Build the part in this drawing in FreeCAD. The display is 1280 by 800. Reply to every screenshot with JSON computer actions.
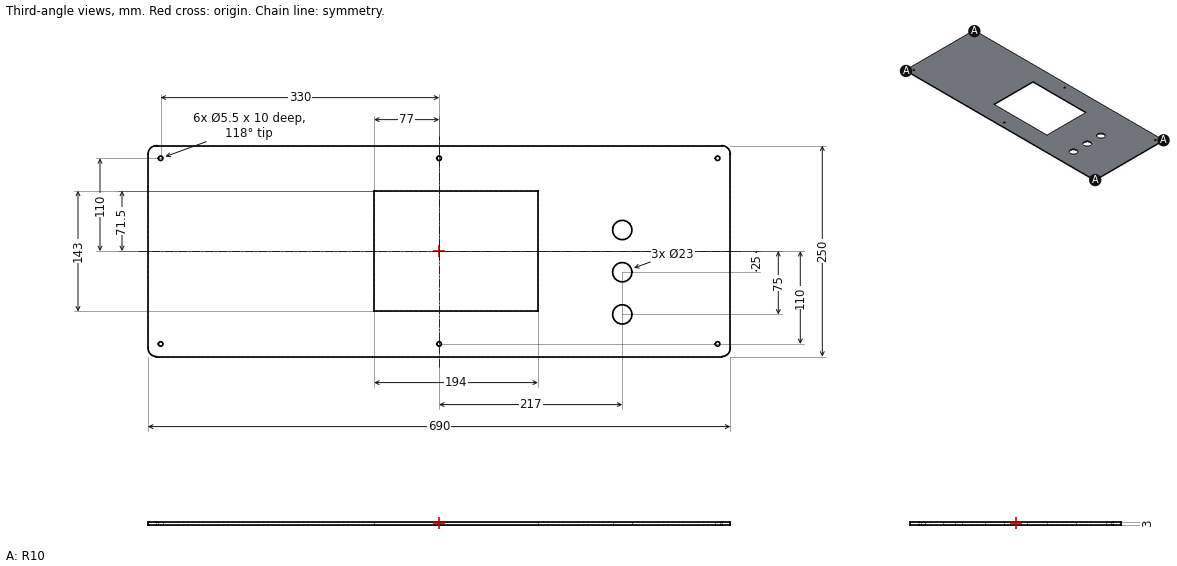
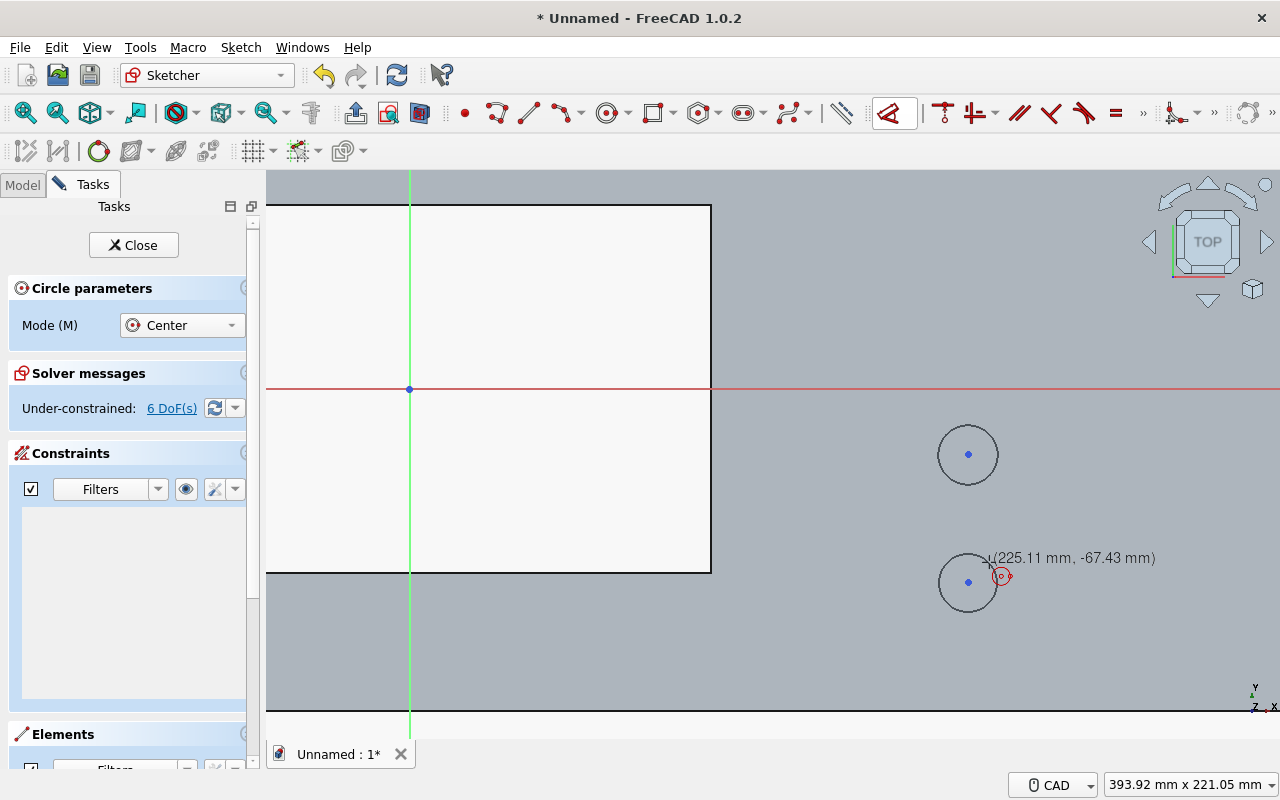
{"action": "left_click", "coordinate": [968, 325]}
{"action": "left_click", "coordinate": [989, 304]}
{"action": "key", "text": "Escape"}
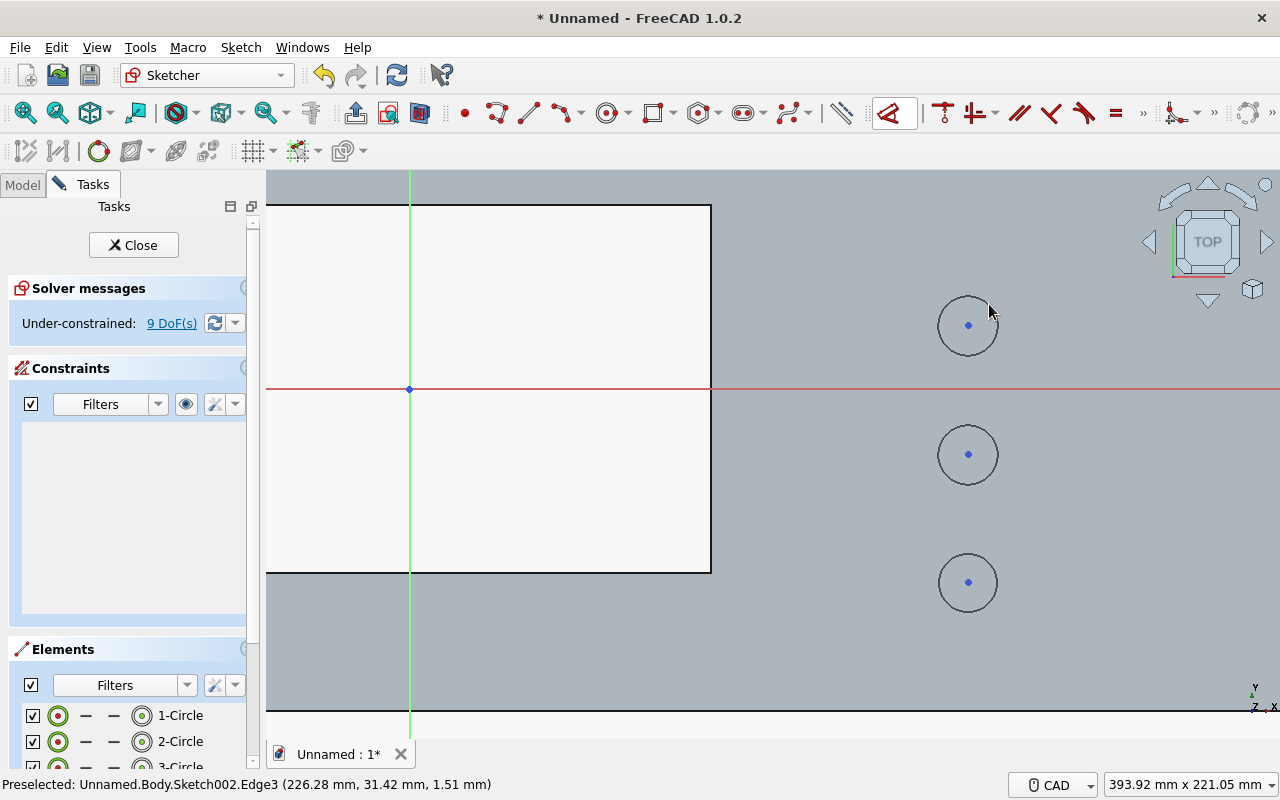
{"action": "left_click", "coordinate": [989, 434]}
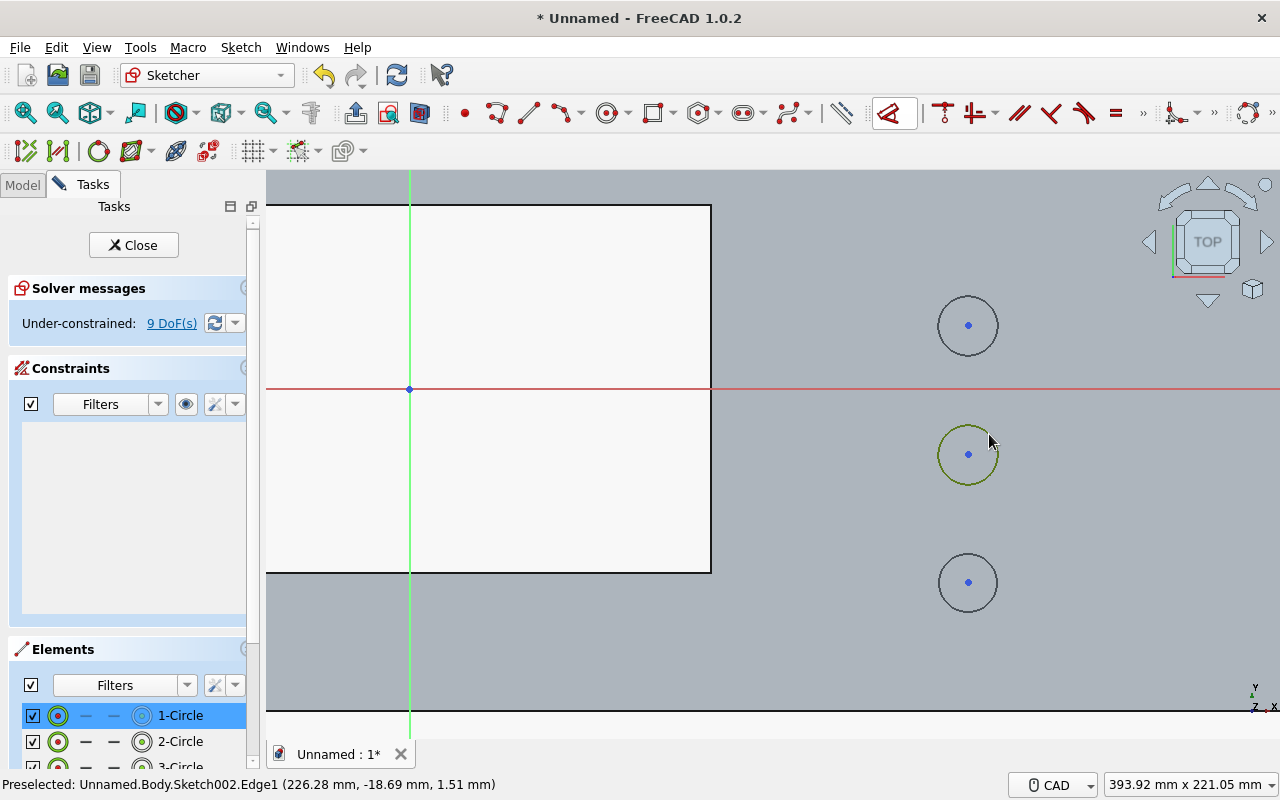
{"action": "left_click", "coordinate": [988, 562]}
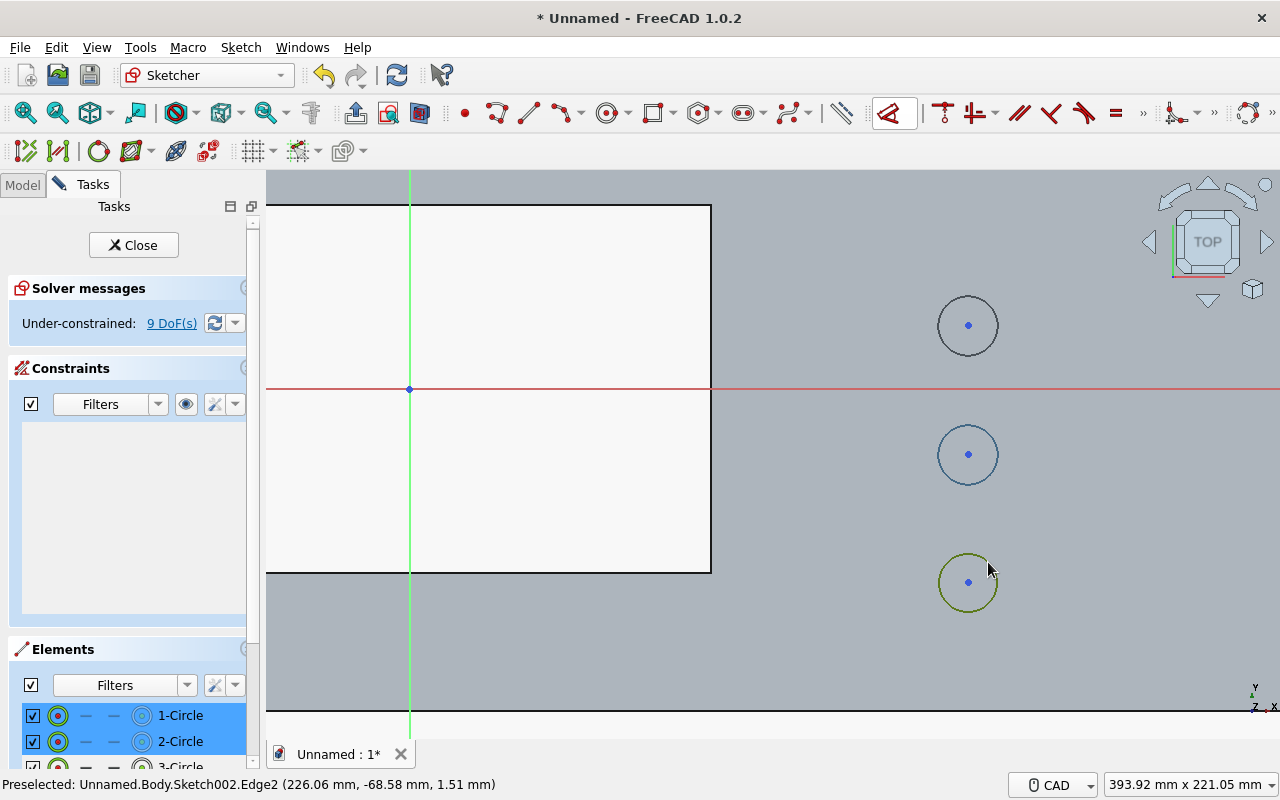
{"action": "left_click", "coordinate": [989, 305]}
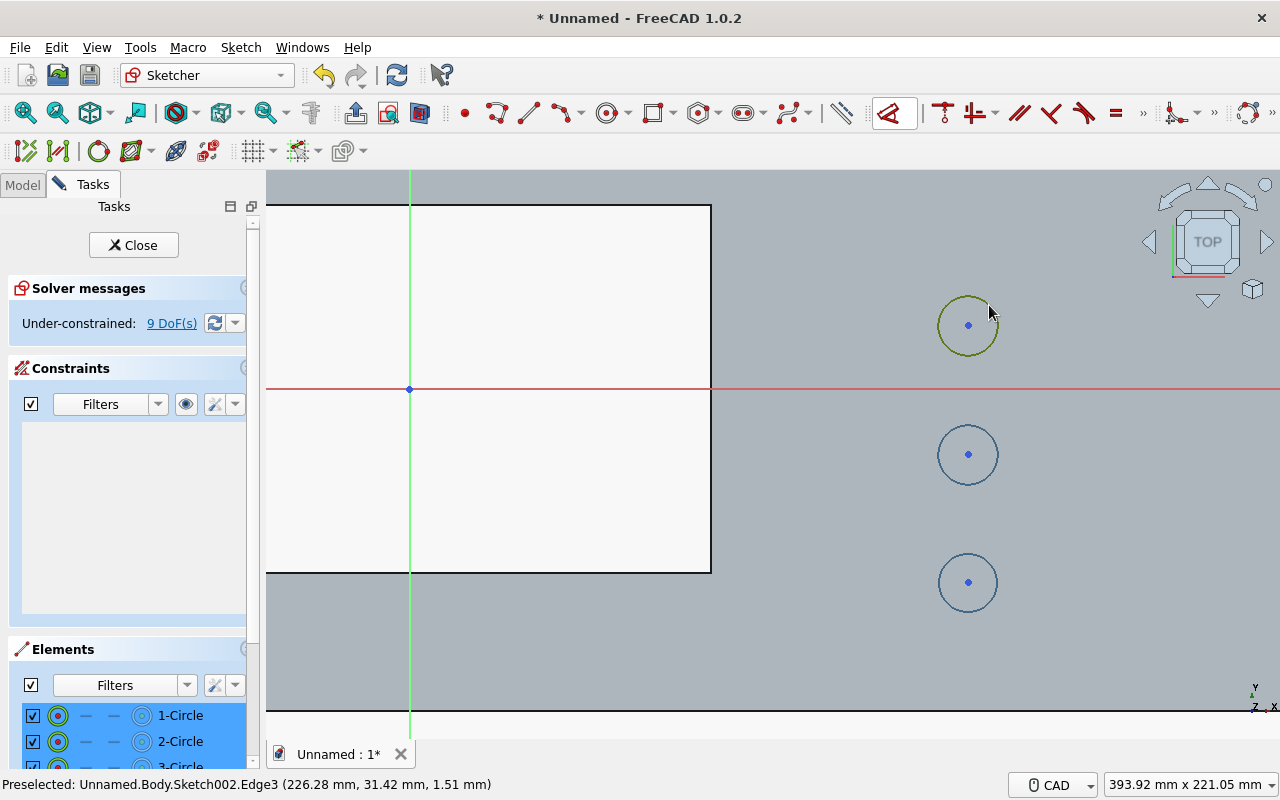
{"action": "left_click", "coordinate": [1116, 114]}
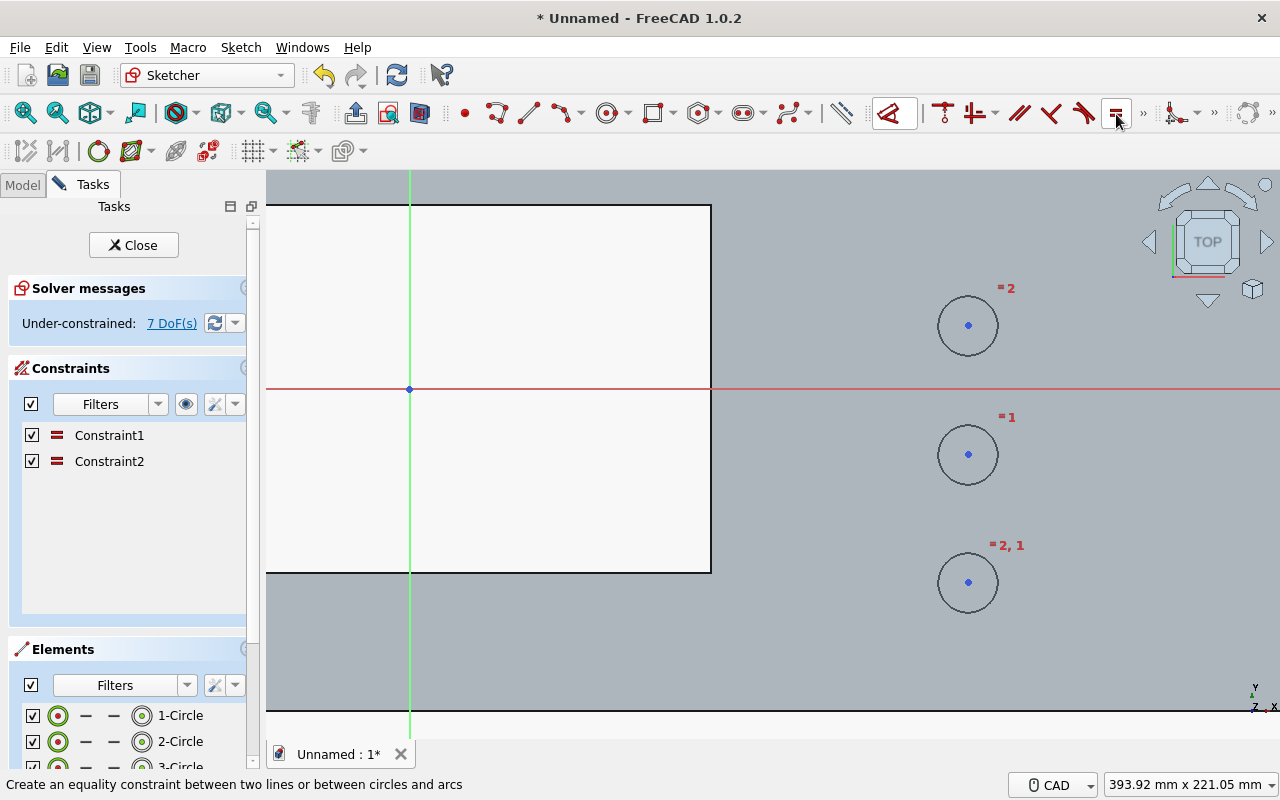
{"action": "left_click", "coordinate": [968, 455]}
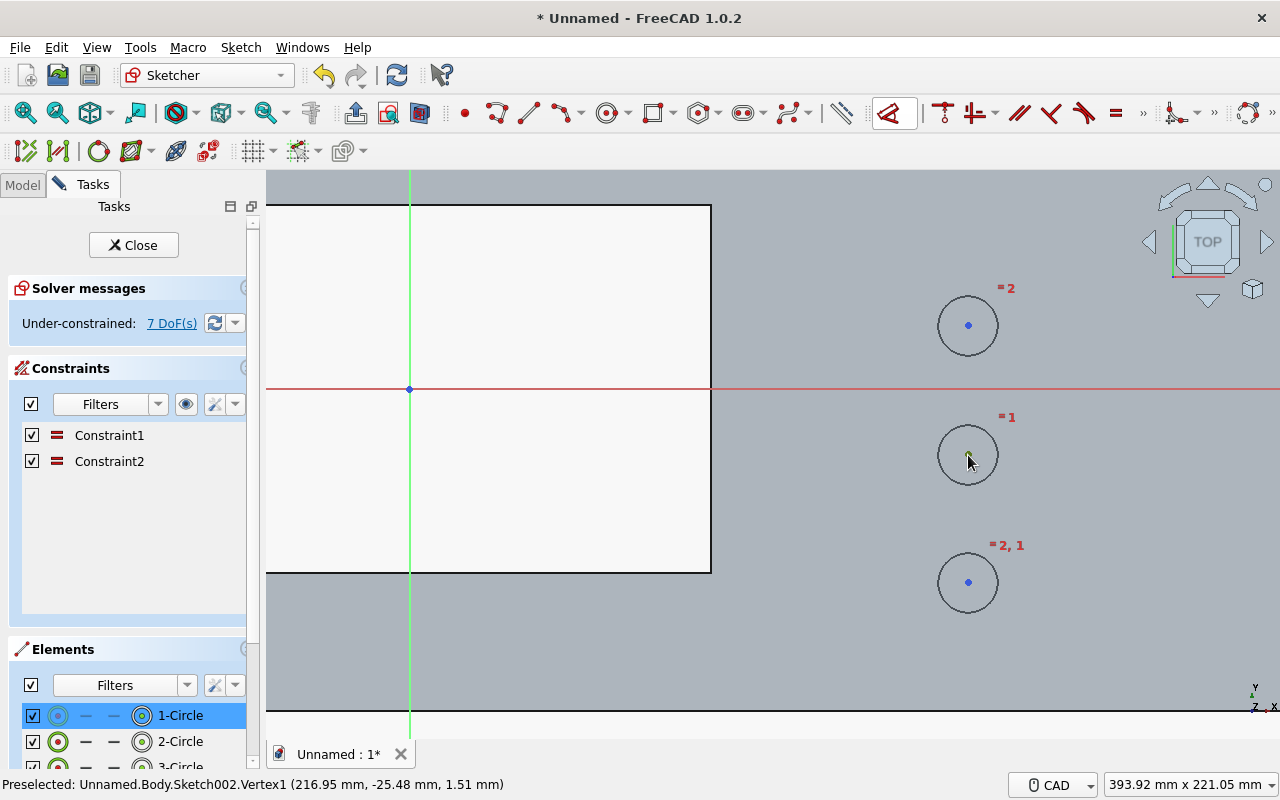
{"action": "left_click", "coordinate": [968, 326]}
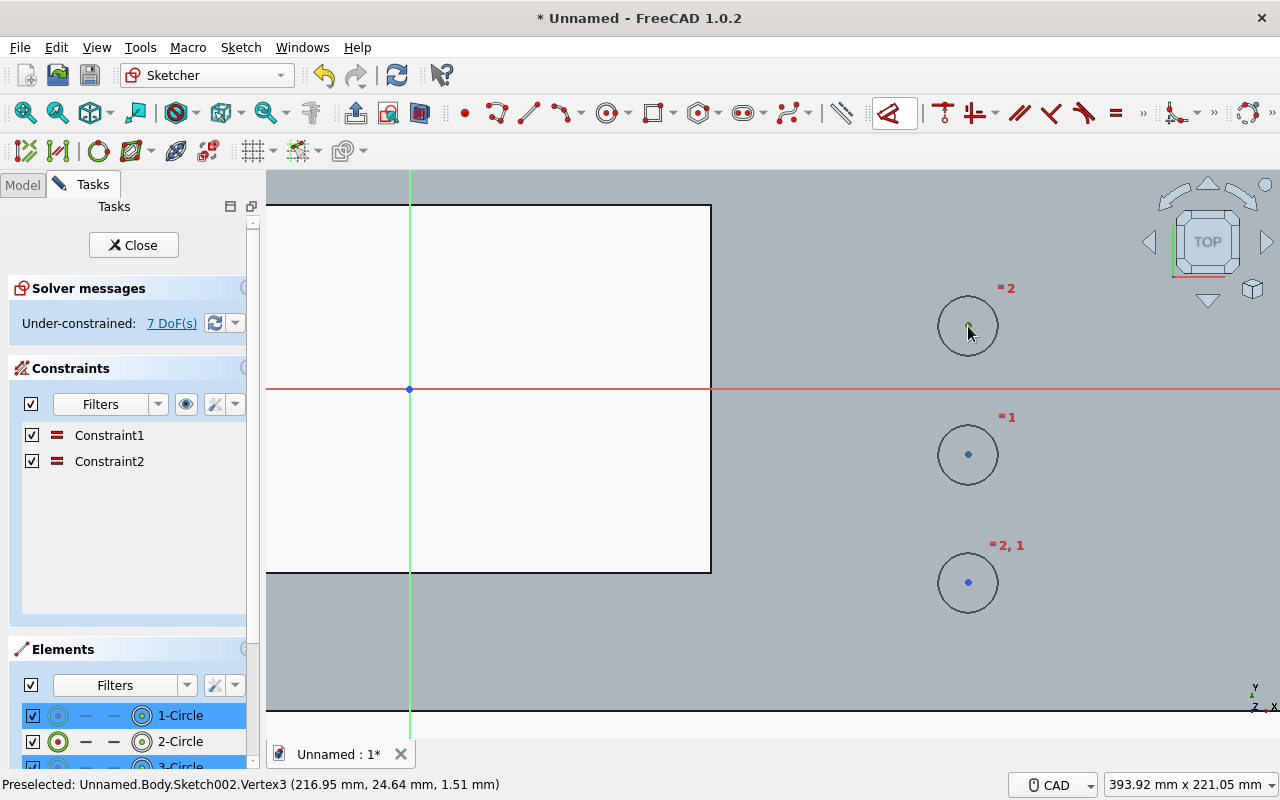
{"action": "left_click", "coordinate": [353, 389]}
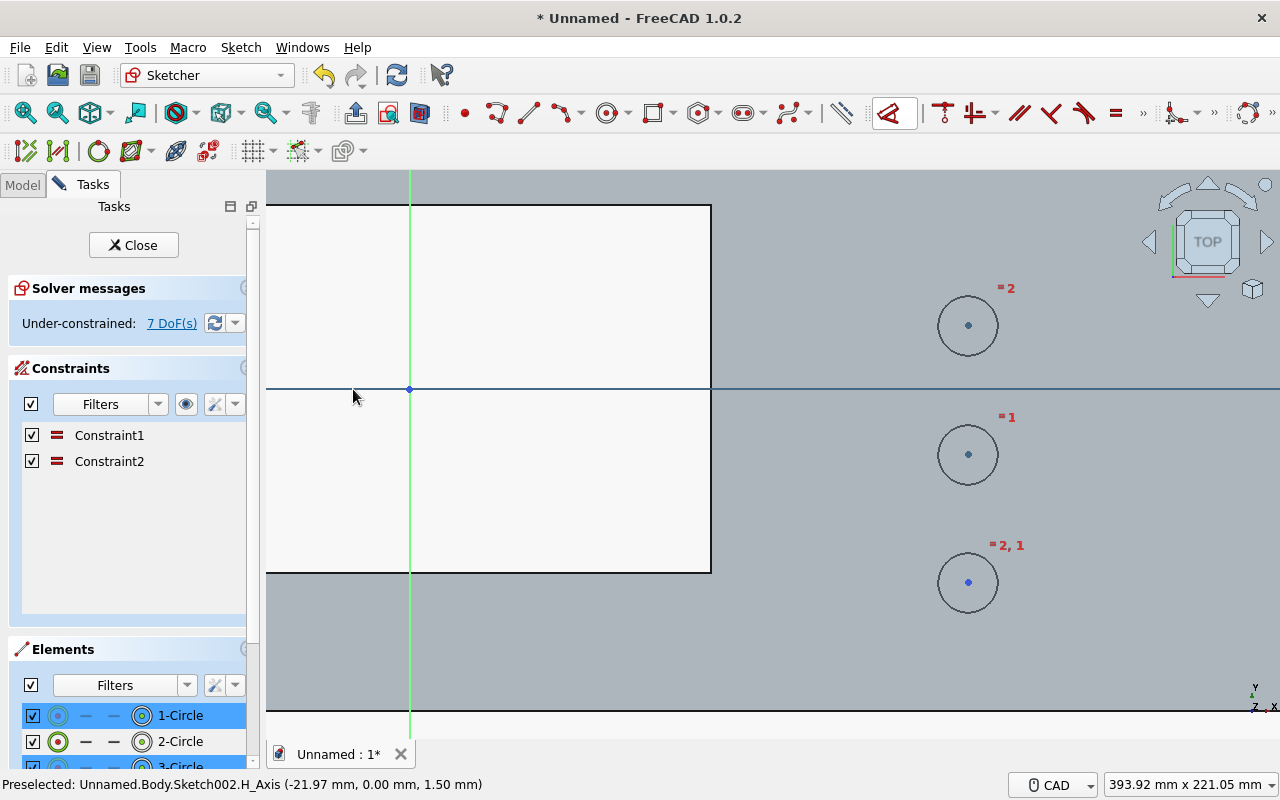
{"action": "key", "text": "s"}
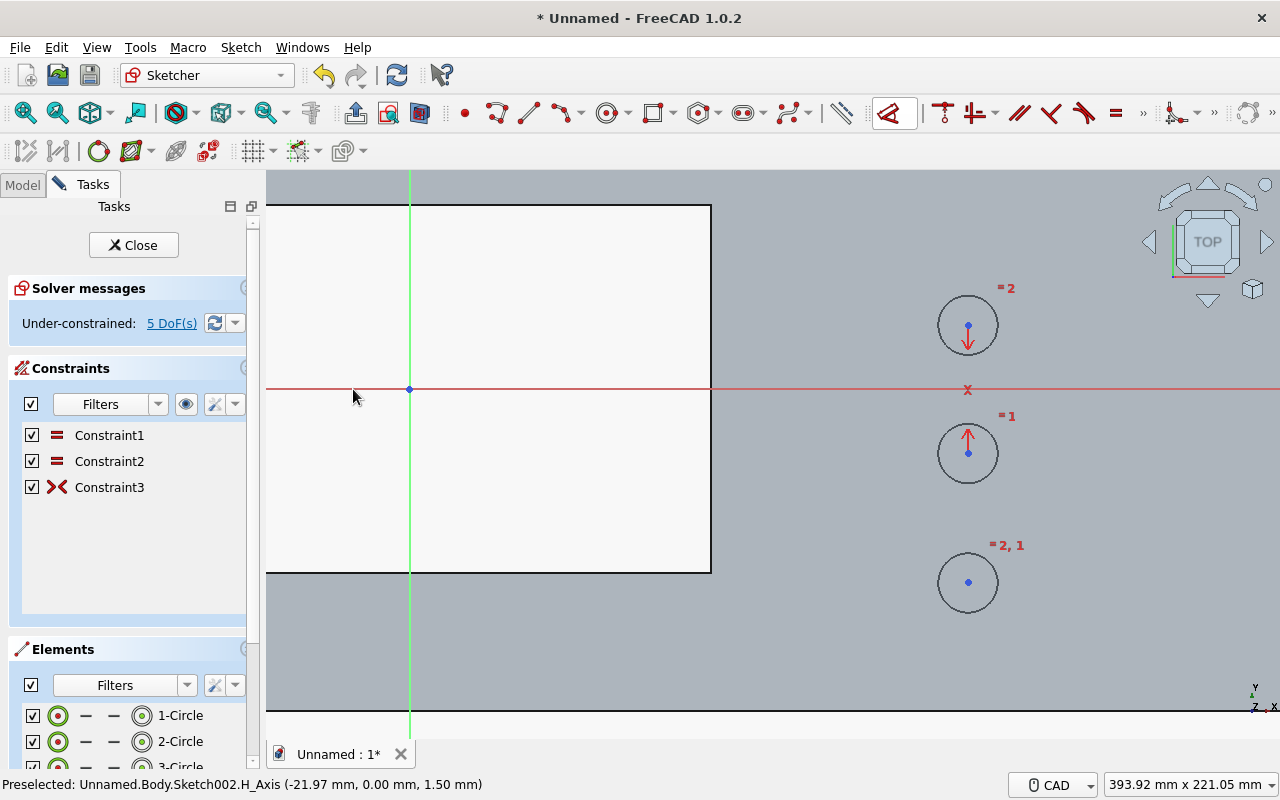
{"action": "left_click", "coordinate": [989, 433]}